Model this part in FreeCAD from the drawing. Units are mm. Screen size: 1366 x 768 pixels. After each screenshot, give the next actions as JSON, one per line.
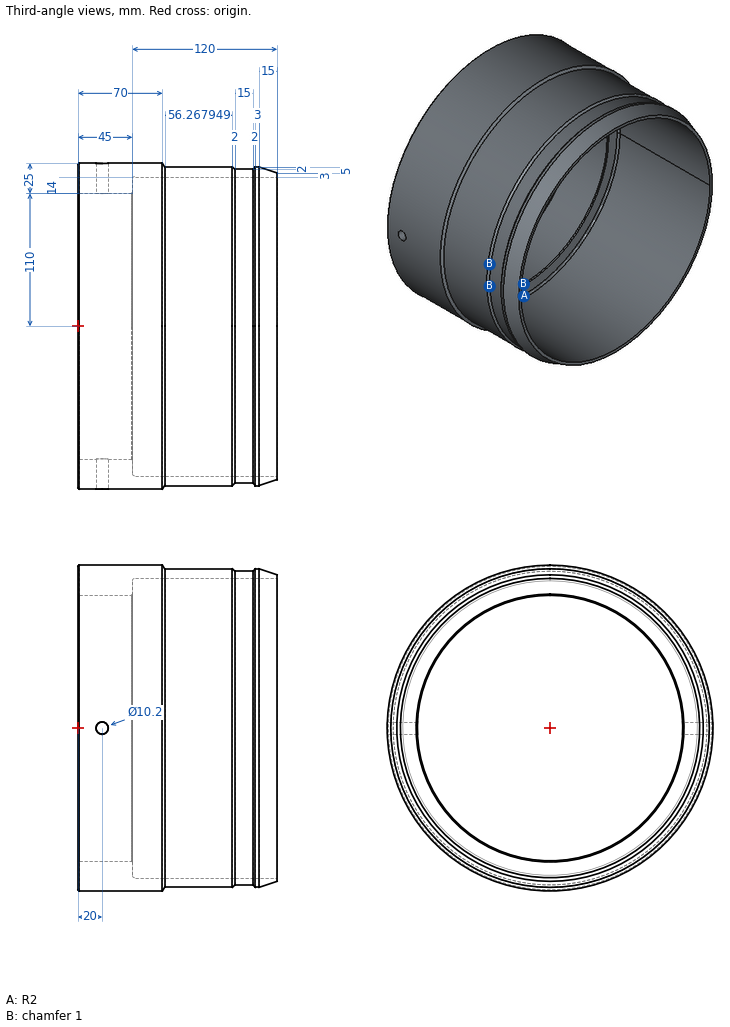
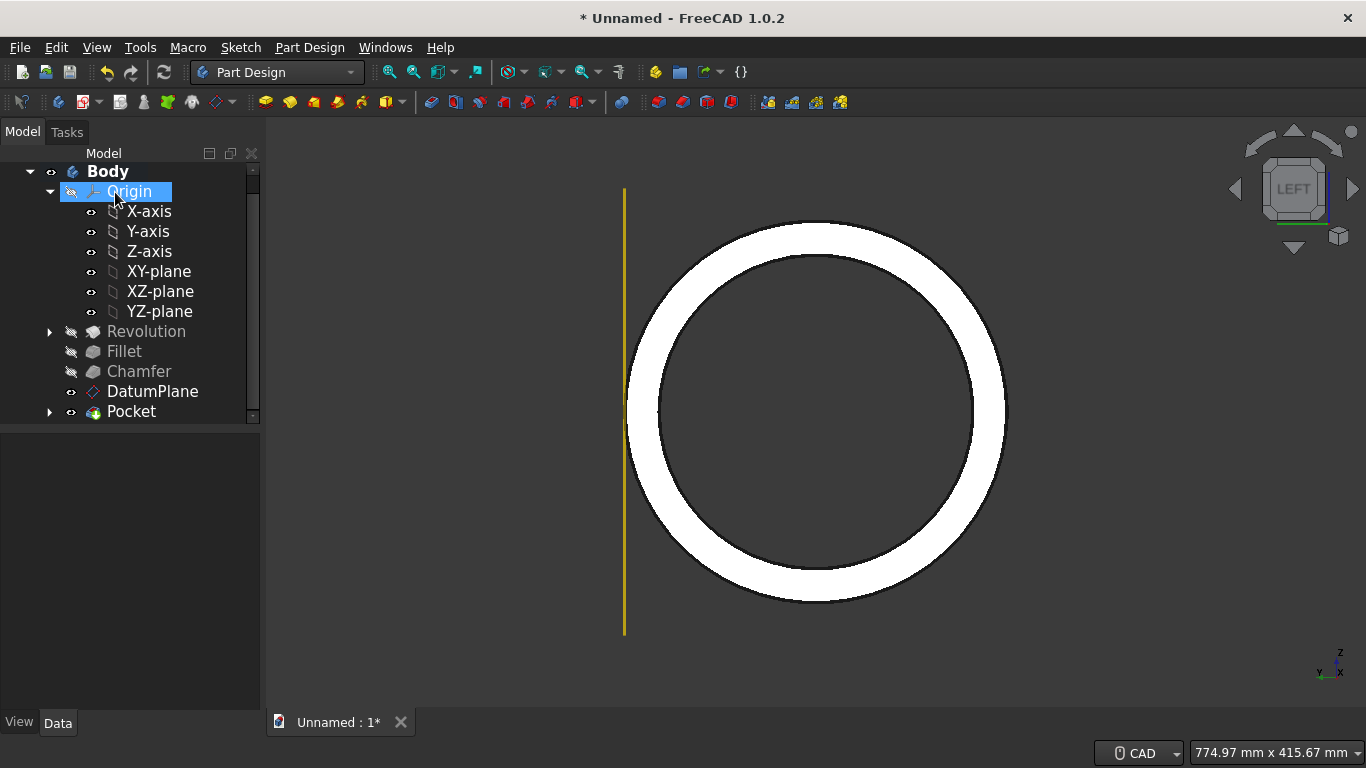
{"action": "left_click", "coordinate": [116, 392]}
{"action": "key", "text": "space"}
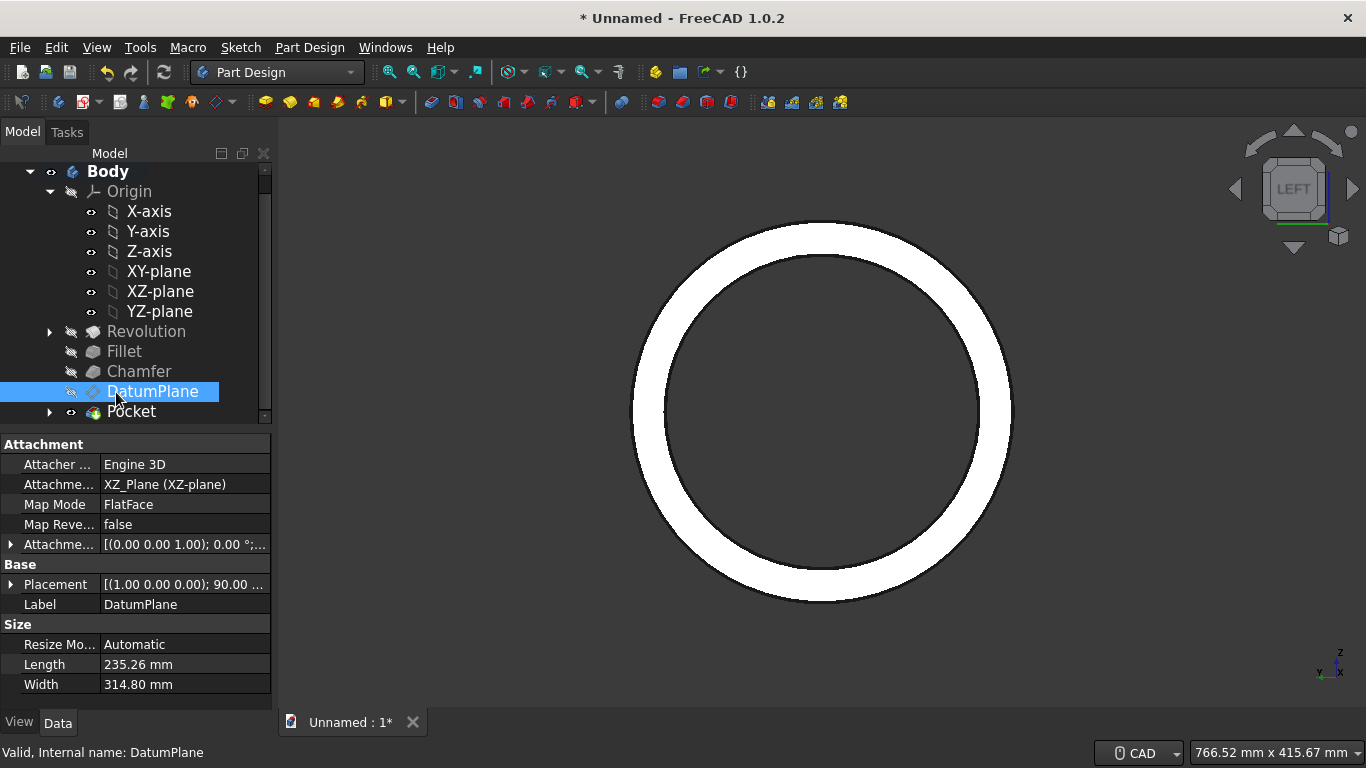
{"action": "key", "text": "0"}